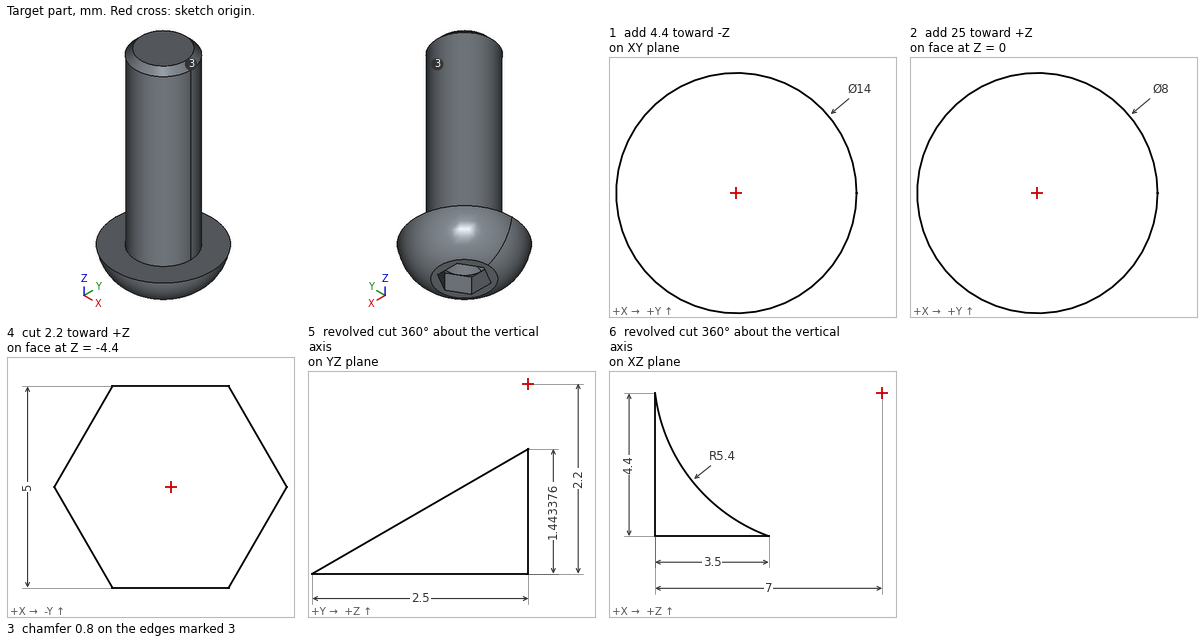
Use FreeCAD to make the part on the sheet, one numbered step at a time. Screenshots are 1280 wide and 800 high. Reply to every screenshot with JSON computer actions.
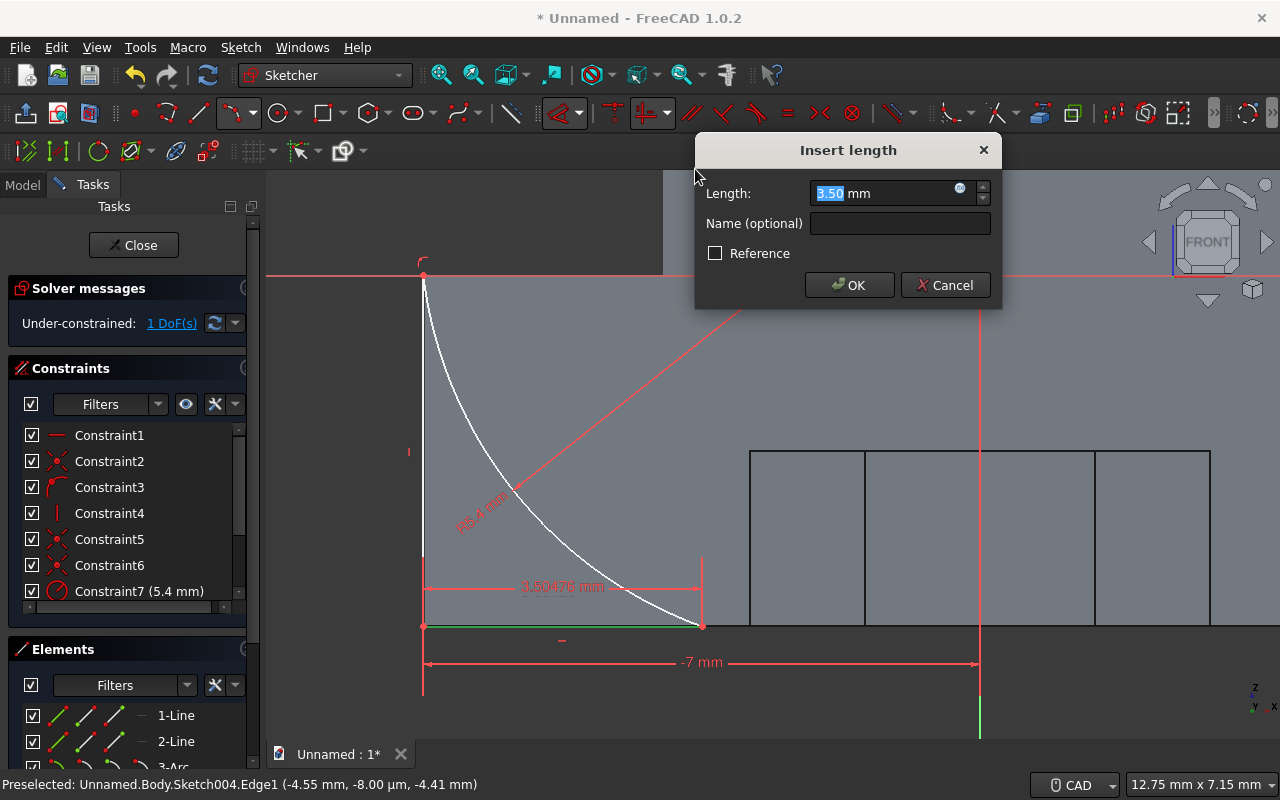
{"action": "type", "text": "3.5"}
{"action": "key", "text": "Return"}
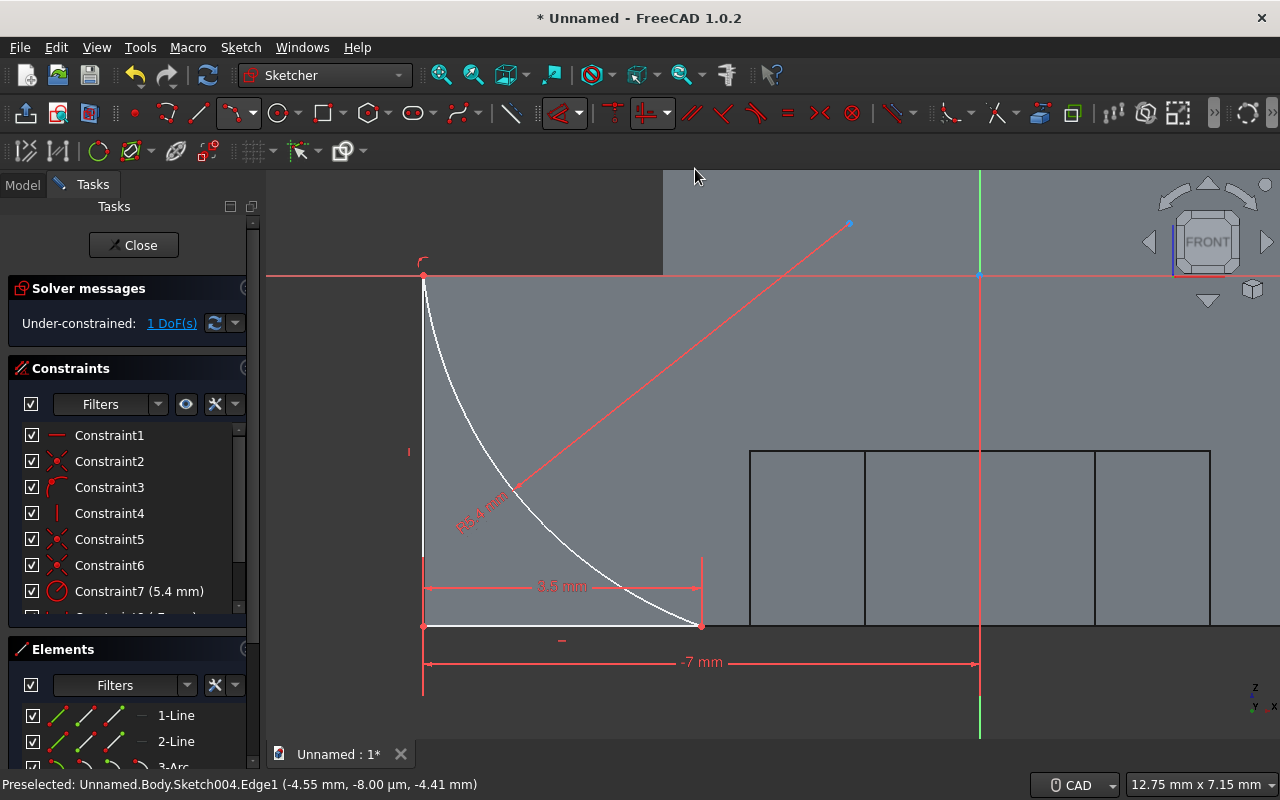
{"action": "left_click", "coordinate": [423, 521]}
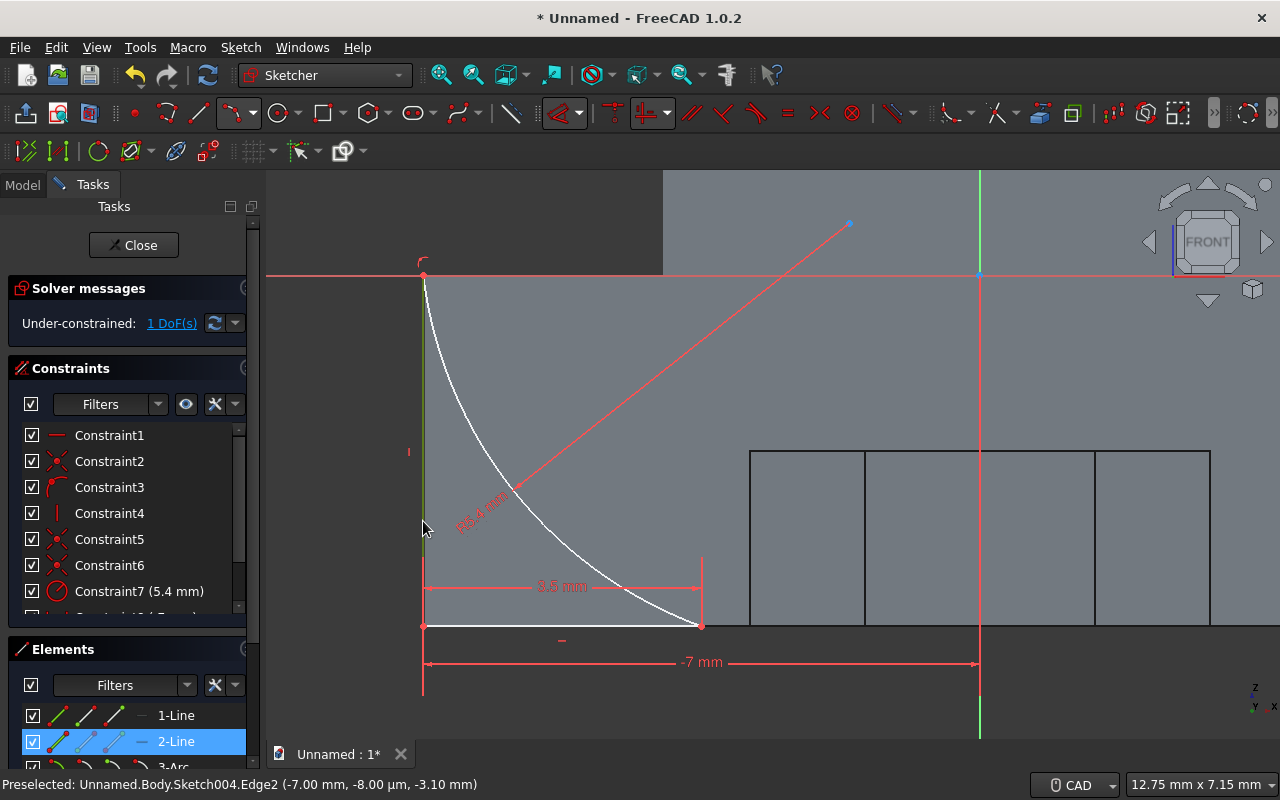
{"action": "key", "text": "i"}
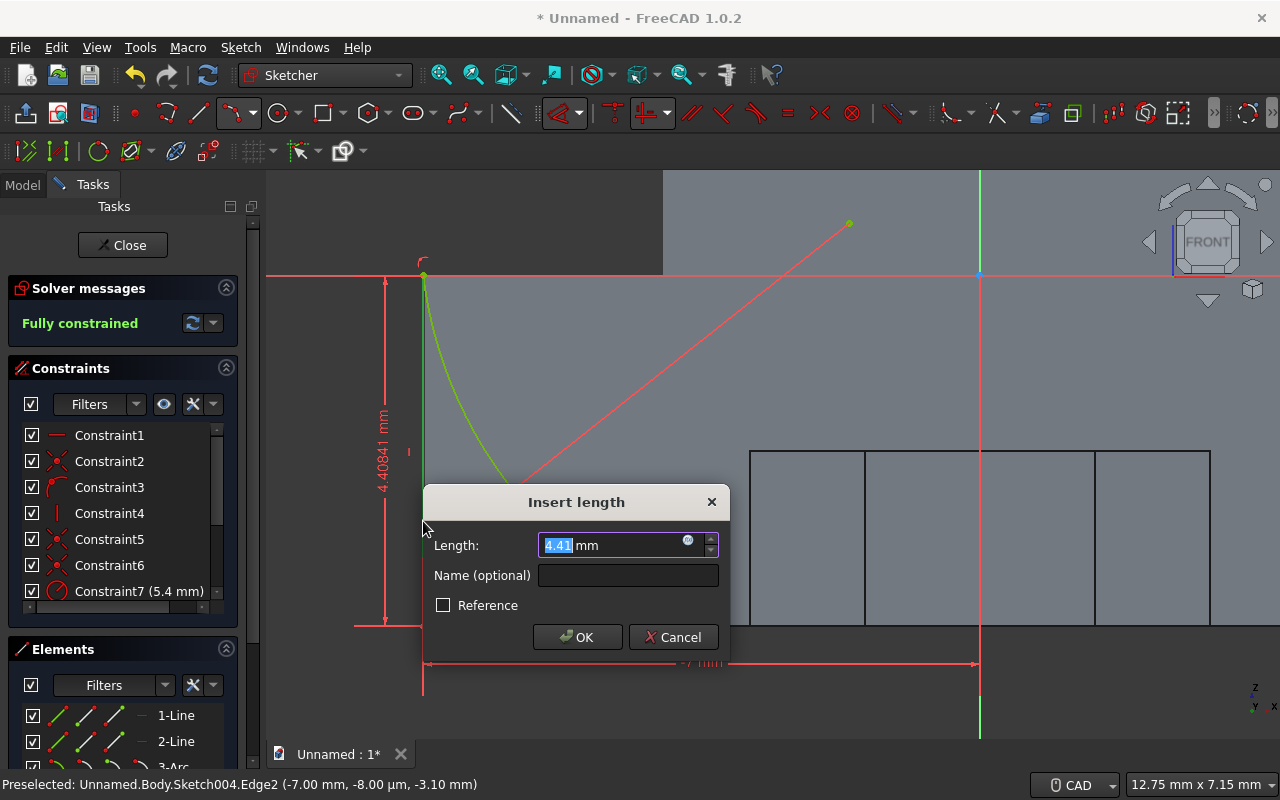
{"action": "type", "text": "4.4"}
{"action": "key", "text": "Return"}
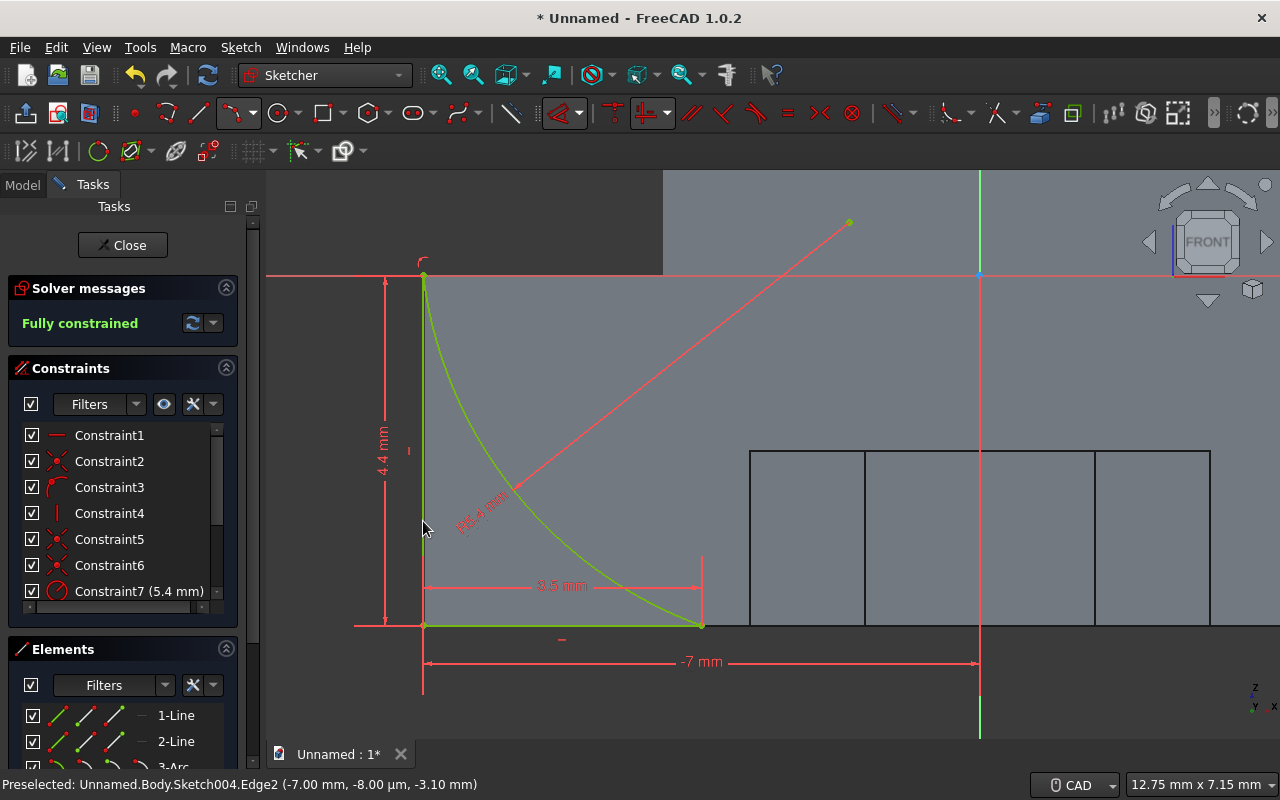
{"action": "left_click", "coordinate": [123, 245]}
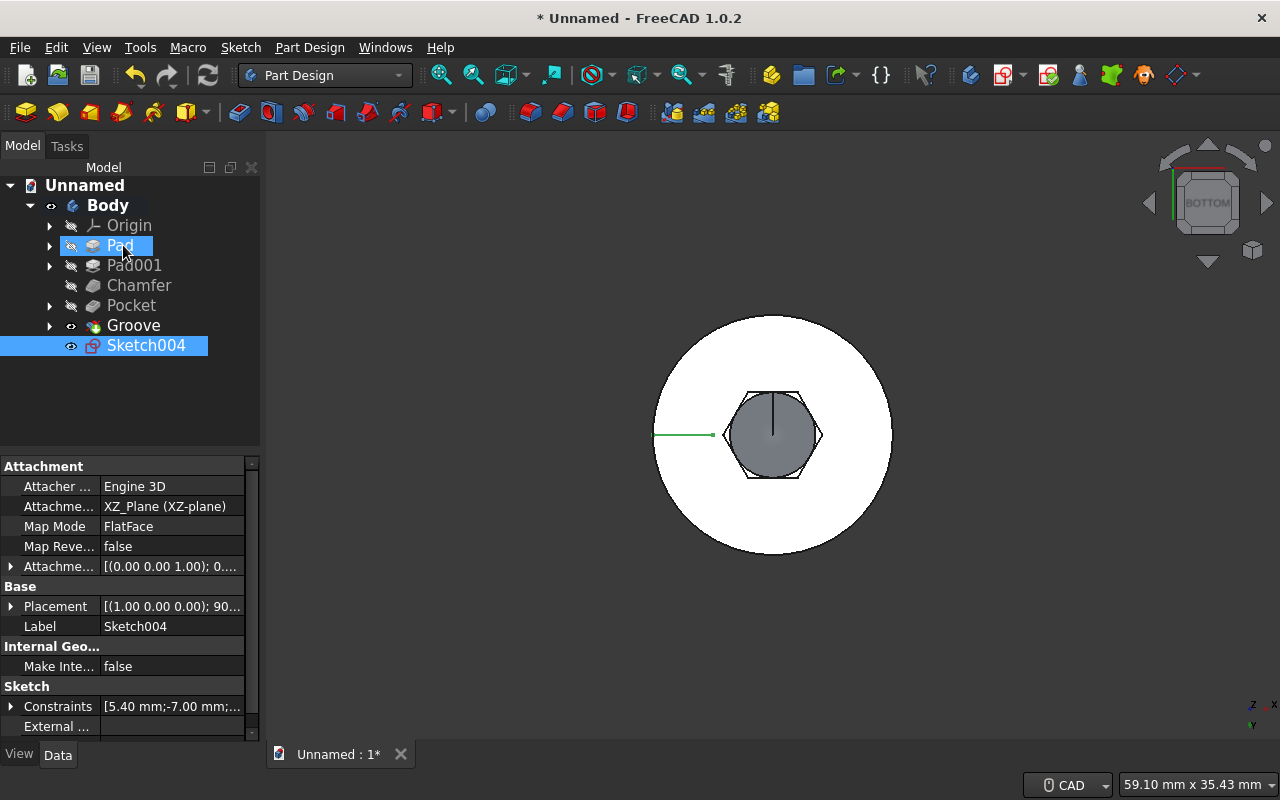
{"action": "left_click", "coordinate": [304, 112]}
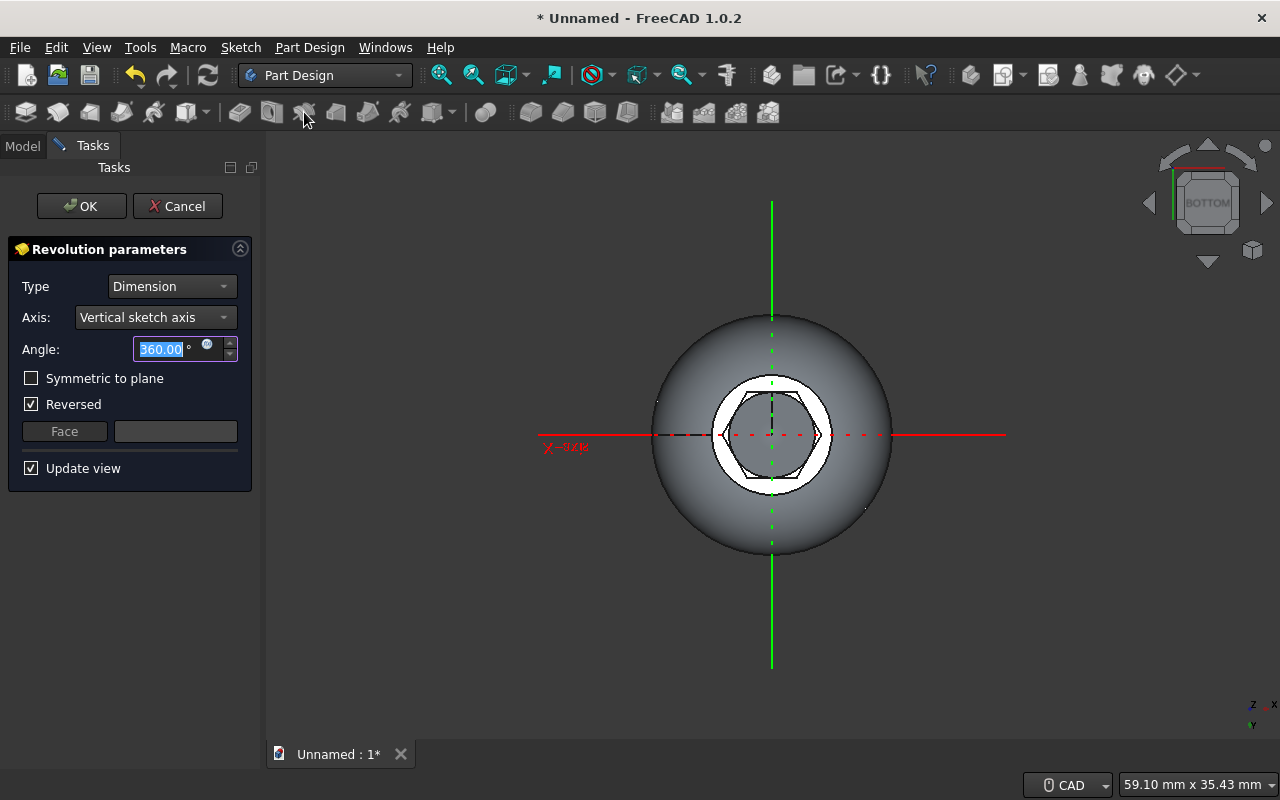
{"action": "left_click", "coordinate": [82, 206]}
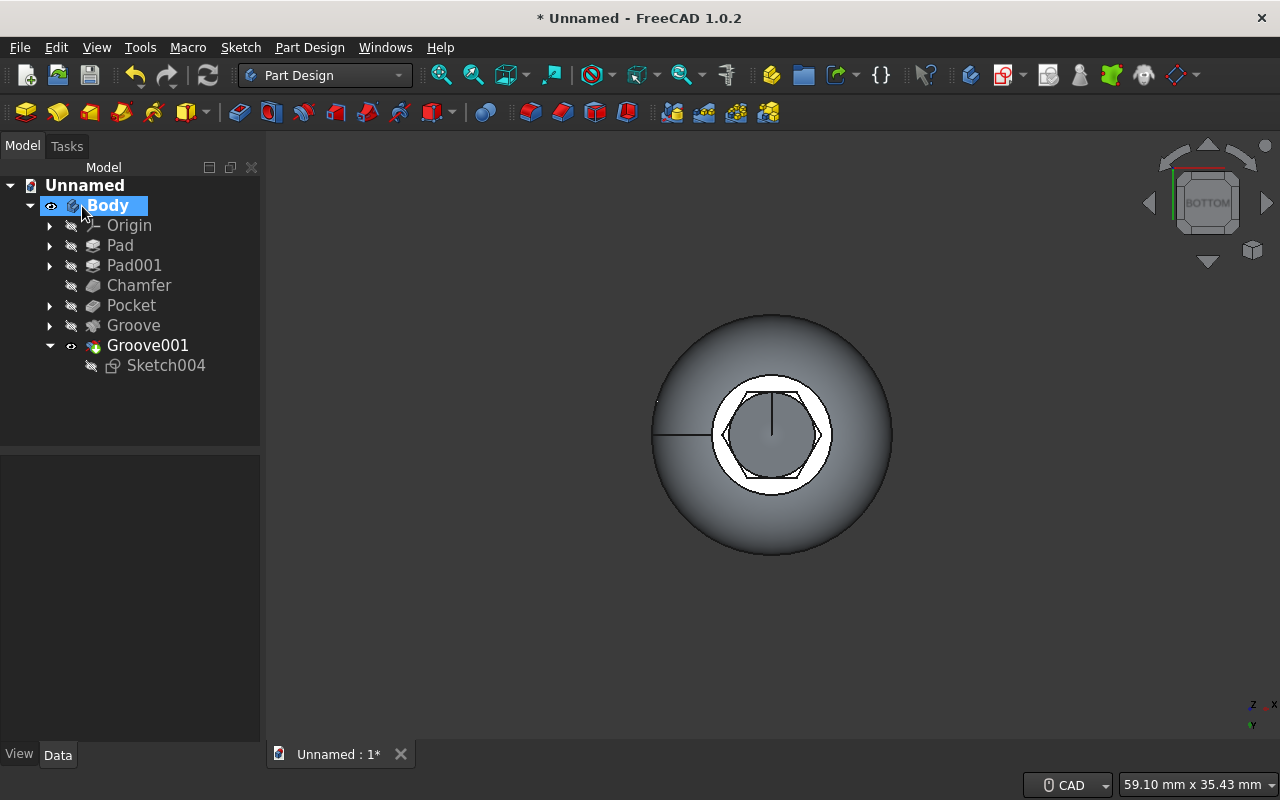
{"action": "key", "text": "0"}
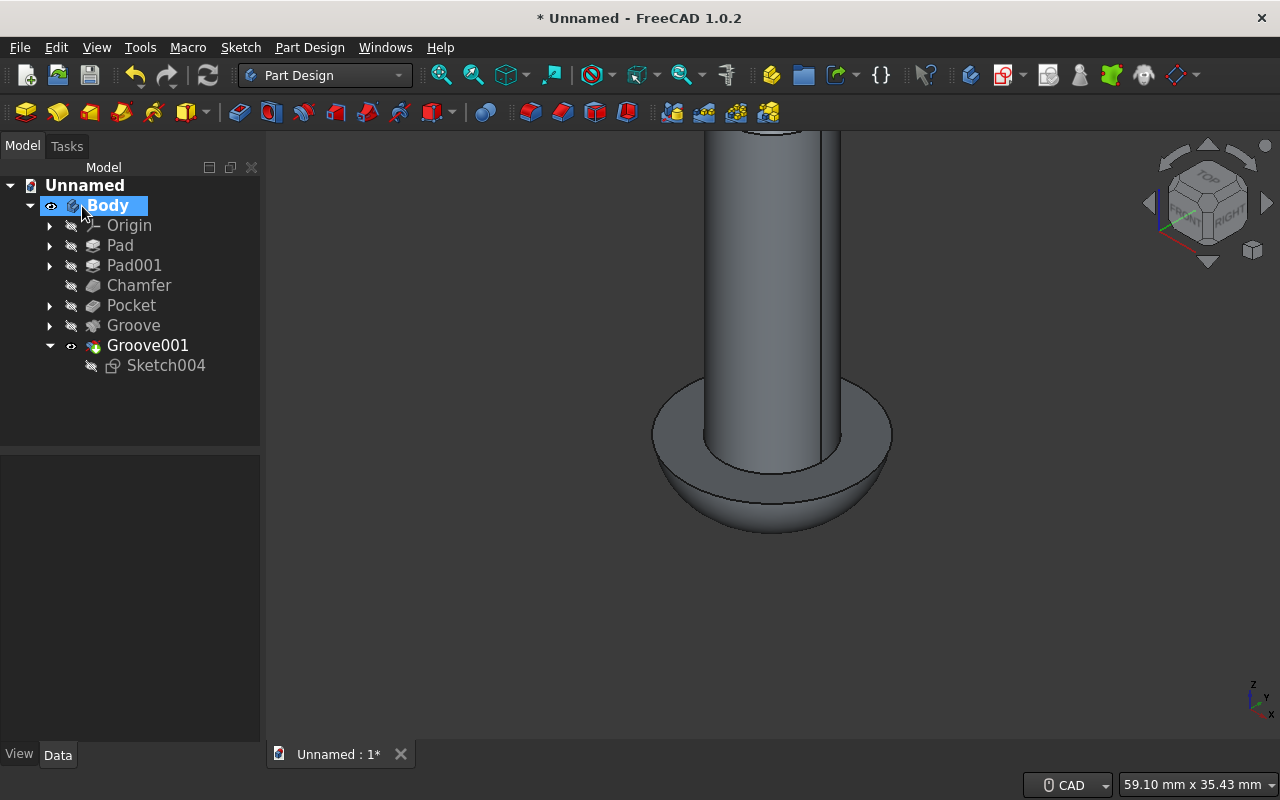
{"action": "left_click", "coordinate": [442, 76]}